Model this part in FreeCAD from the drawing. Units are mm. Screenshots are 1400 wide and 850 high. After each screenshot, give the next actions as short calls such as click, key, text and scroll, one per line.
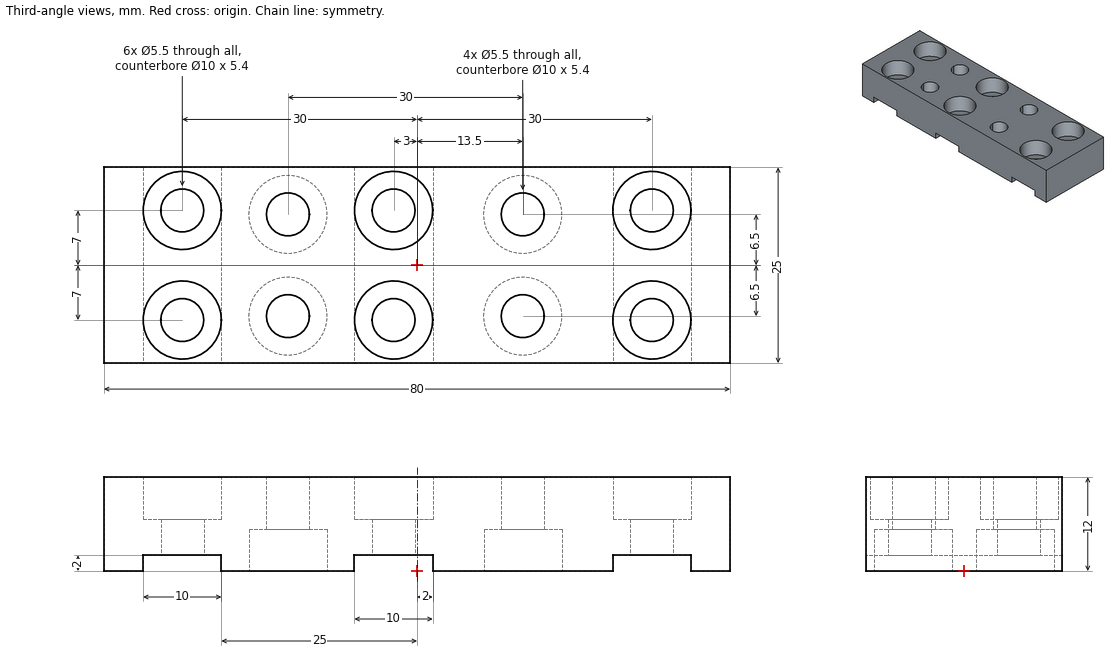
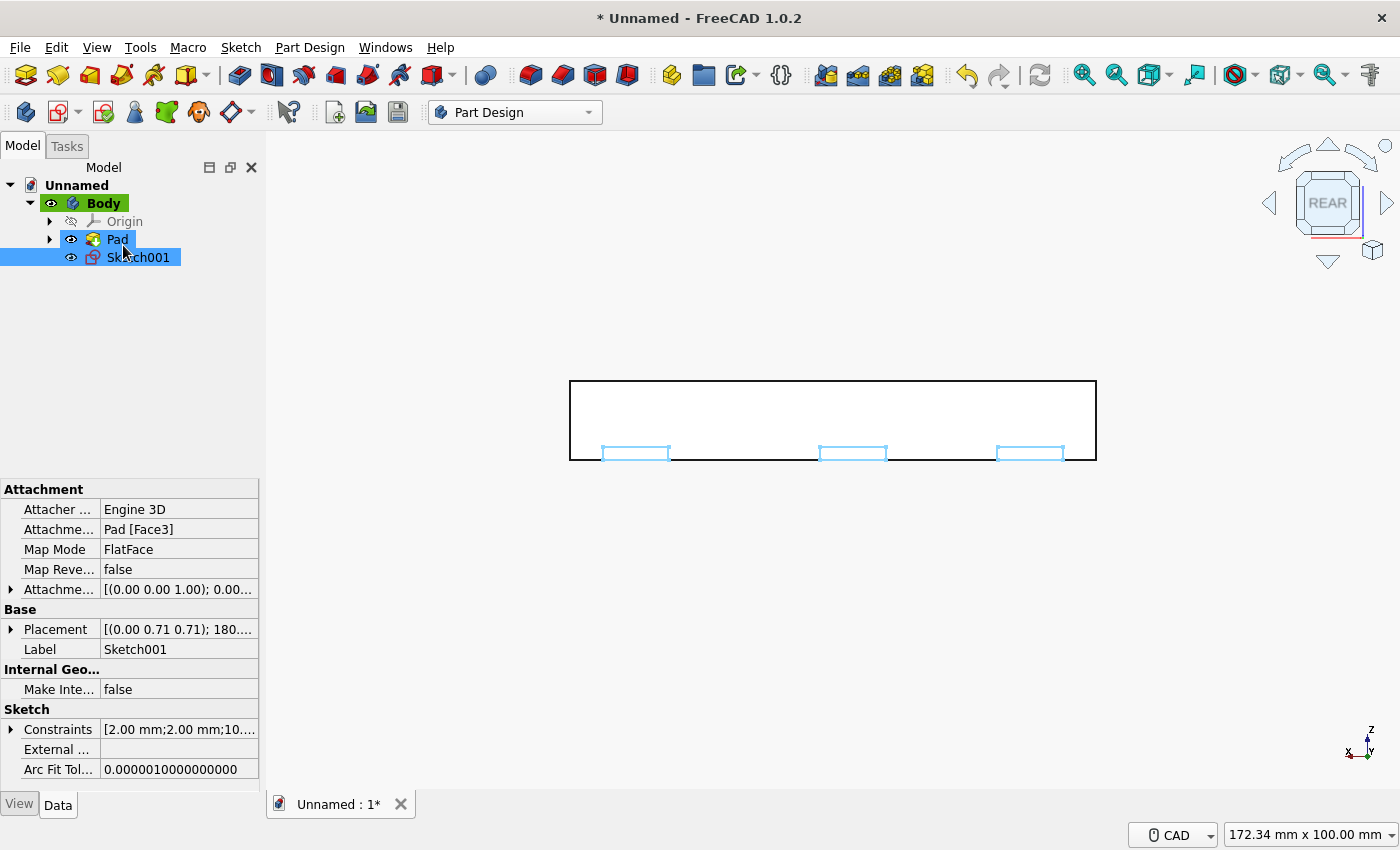
click(240, 76)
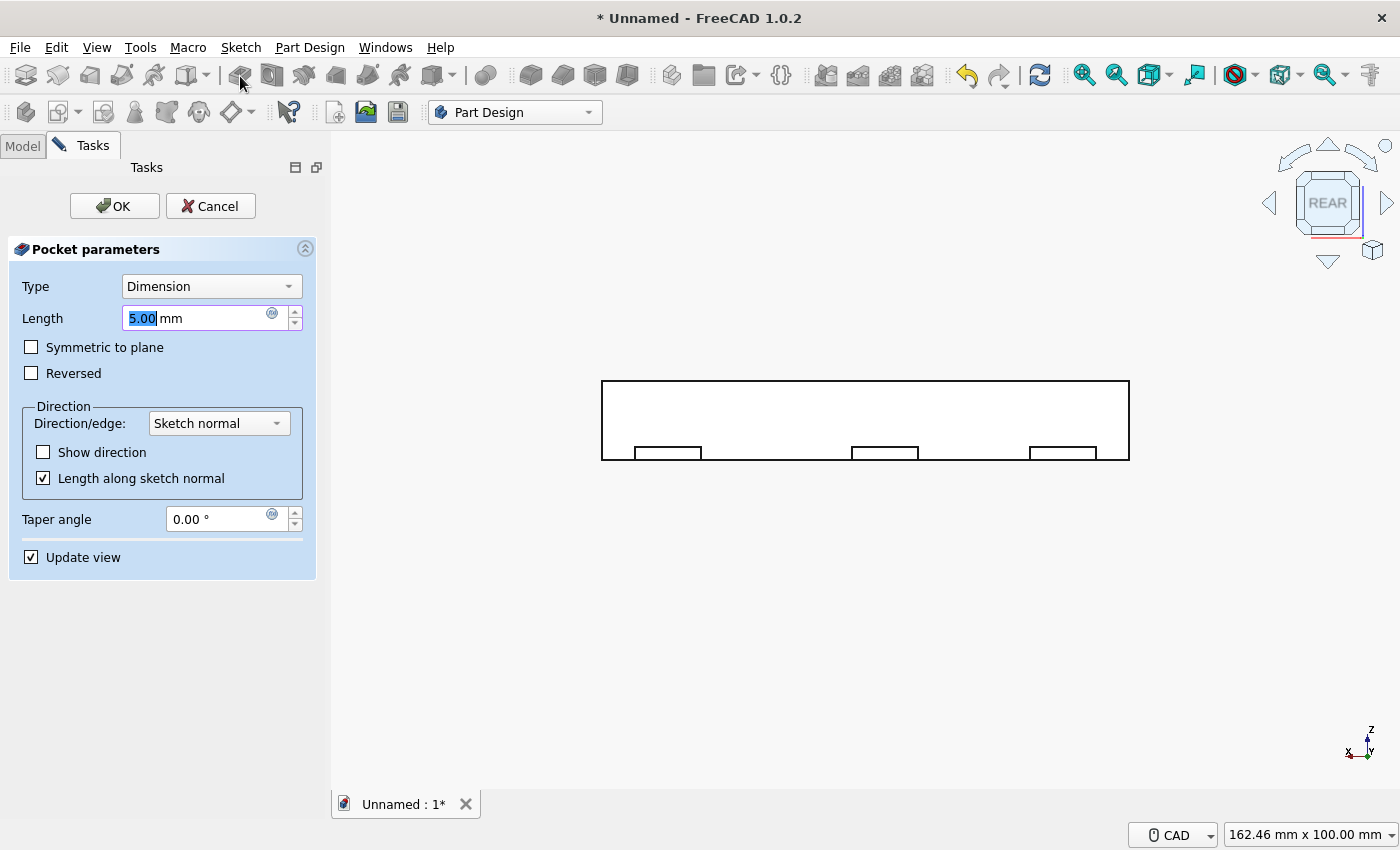
click(212, 286)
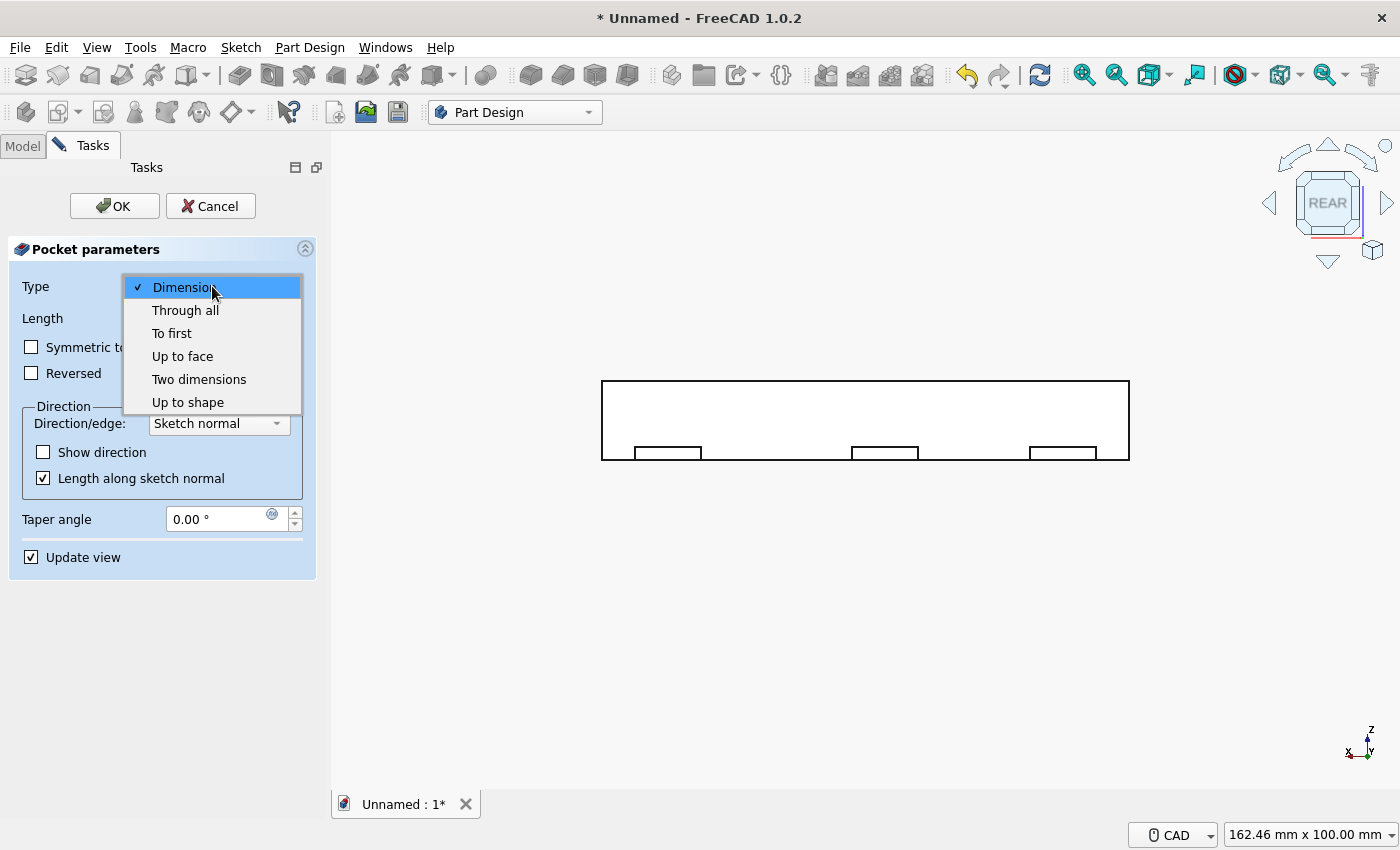
click(212, 310)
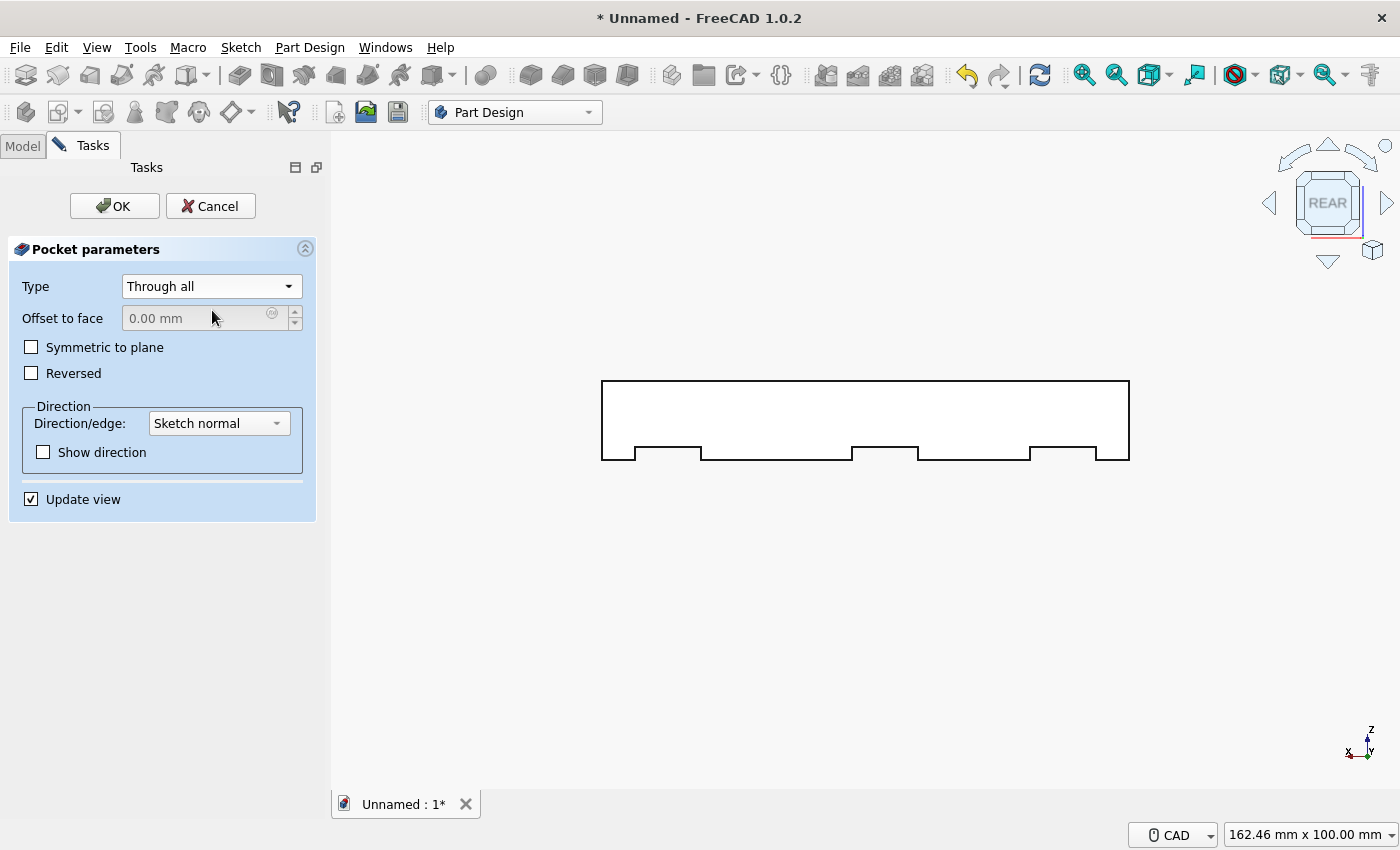
click(115, 206)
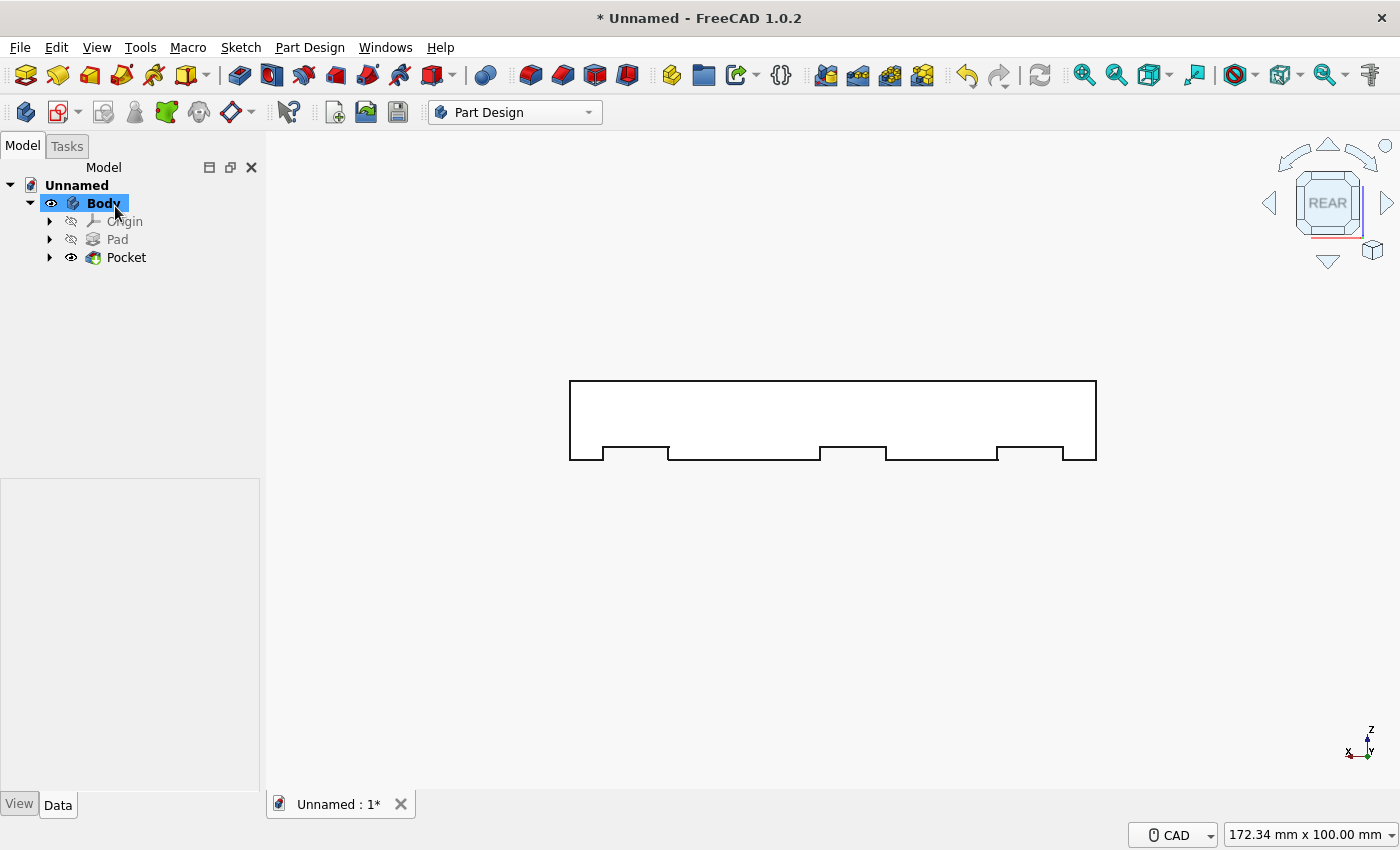
key(0)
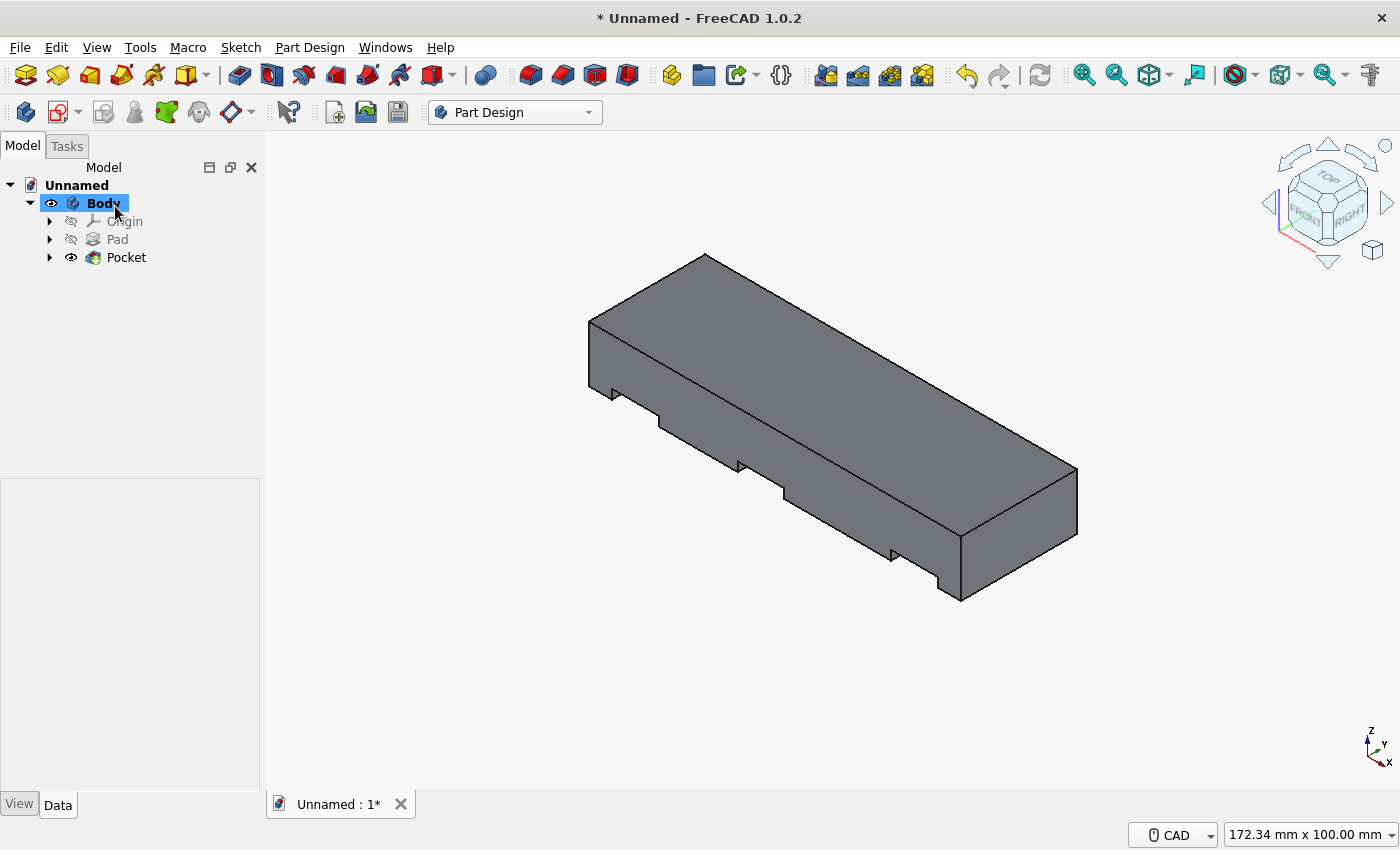
click(939, 456)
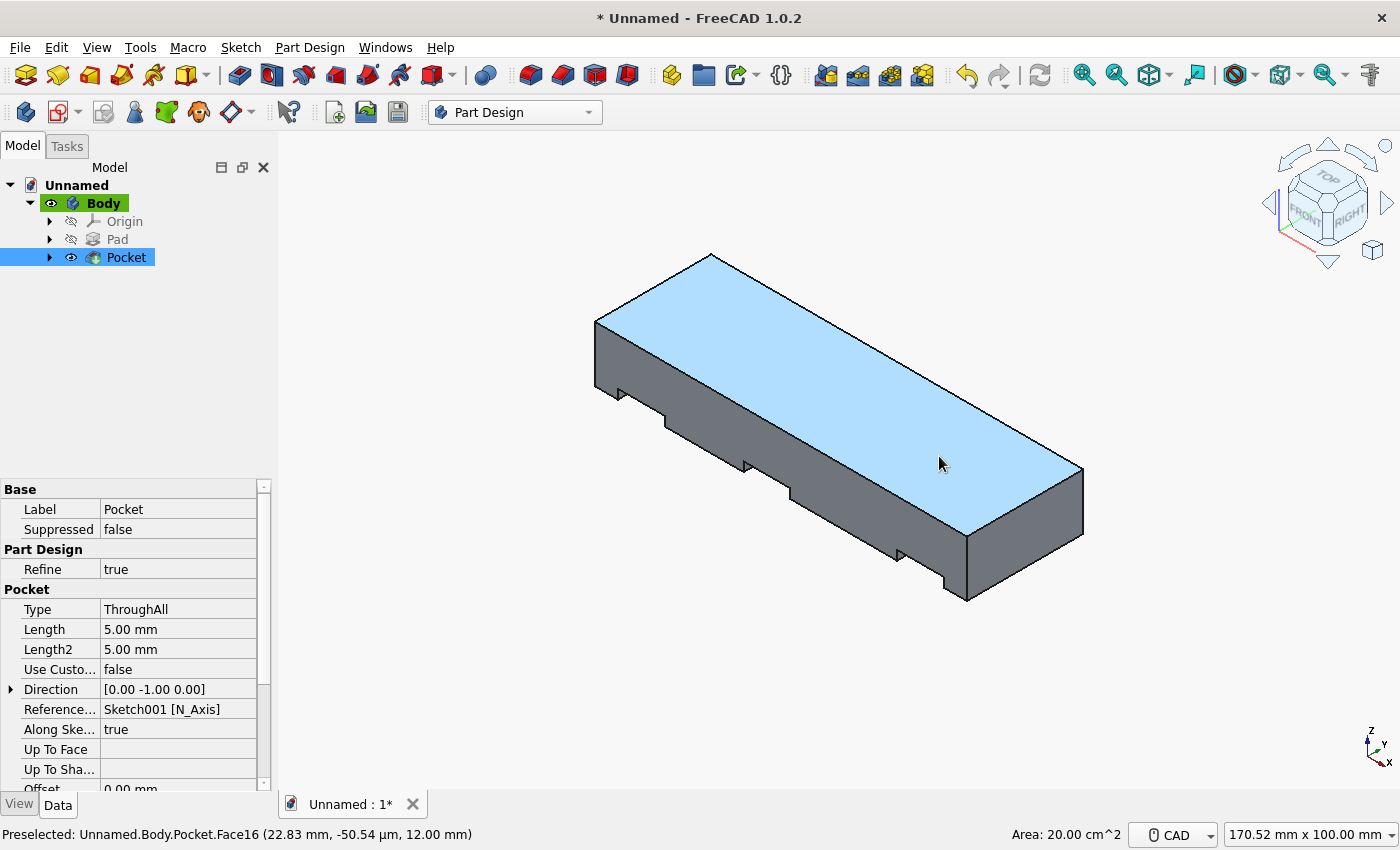
click(58, 112)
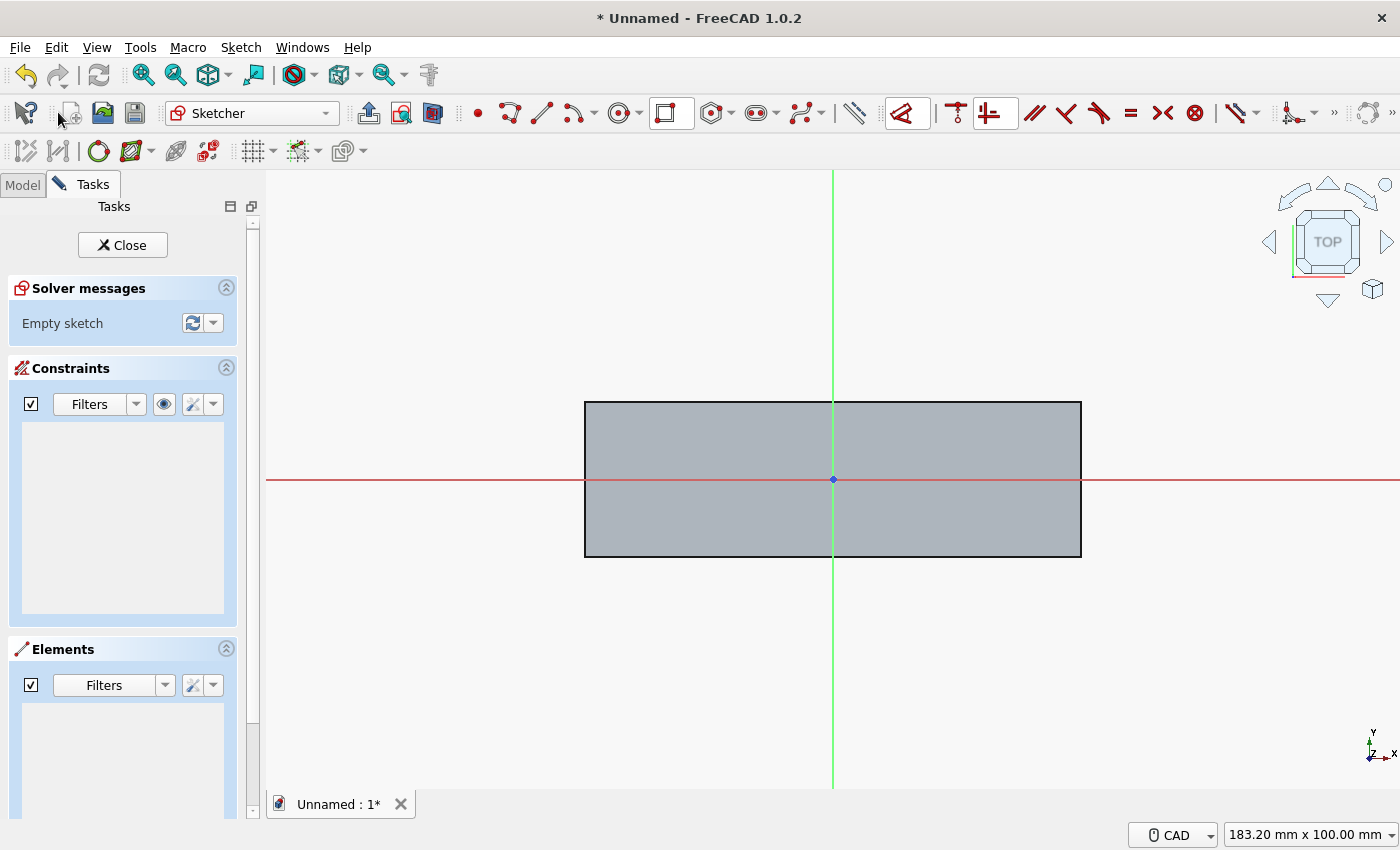
scroll(972, 479, up, 2)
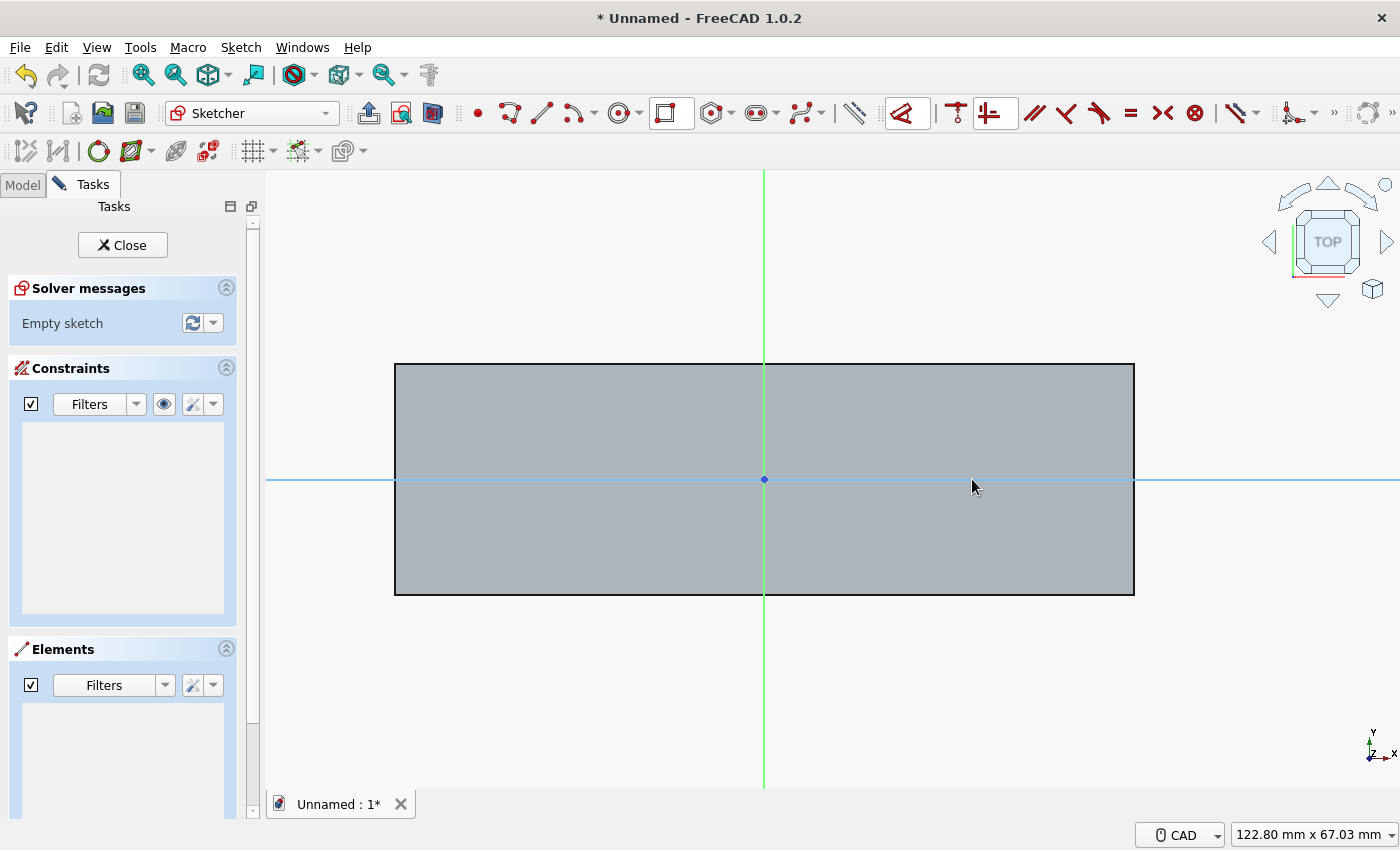
click(620, 114)